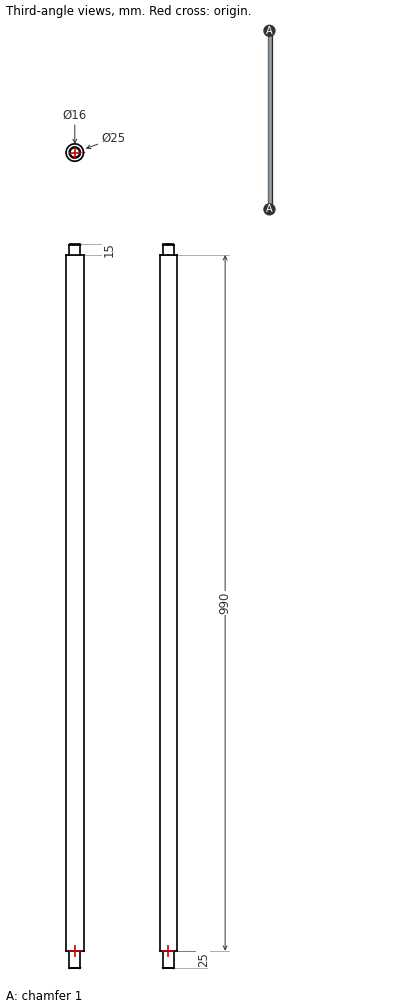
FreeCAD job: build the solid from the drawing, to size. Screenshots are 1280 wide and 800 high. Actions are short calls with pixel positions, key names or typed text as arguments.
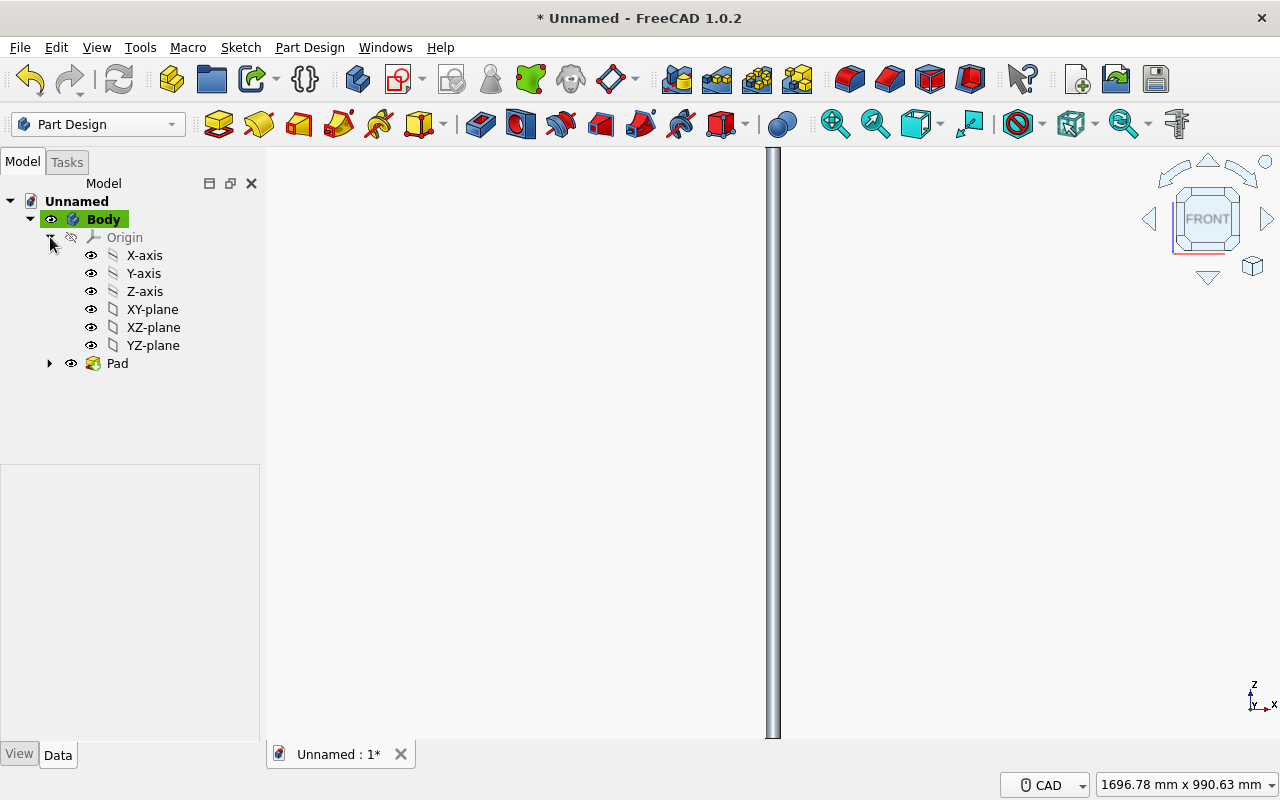
click(136, 309)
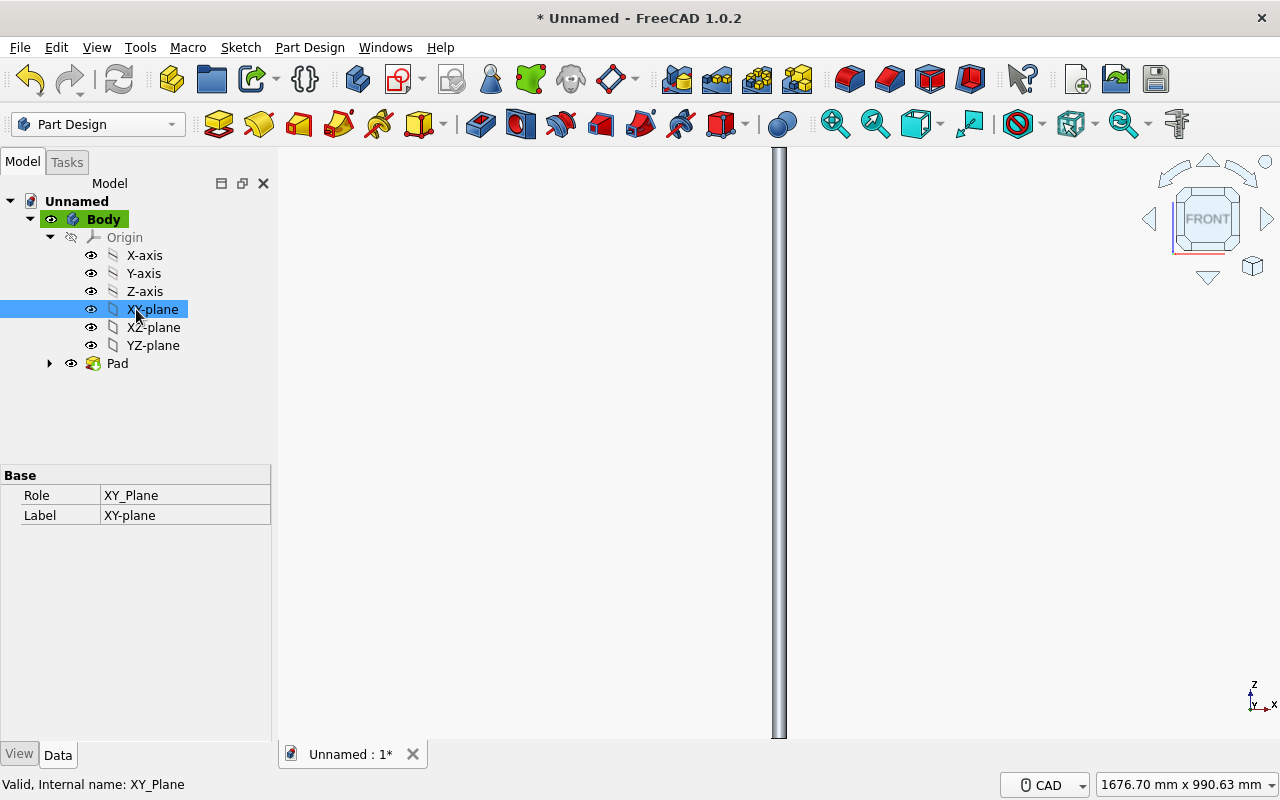
click(612, 80)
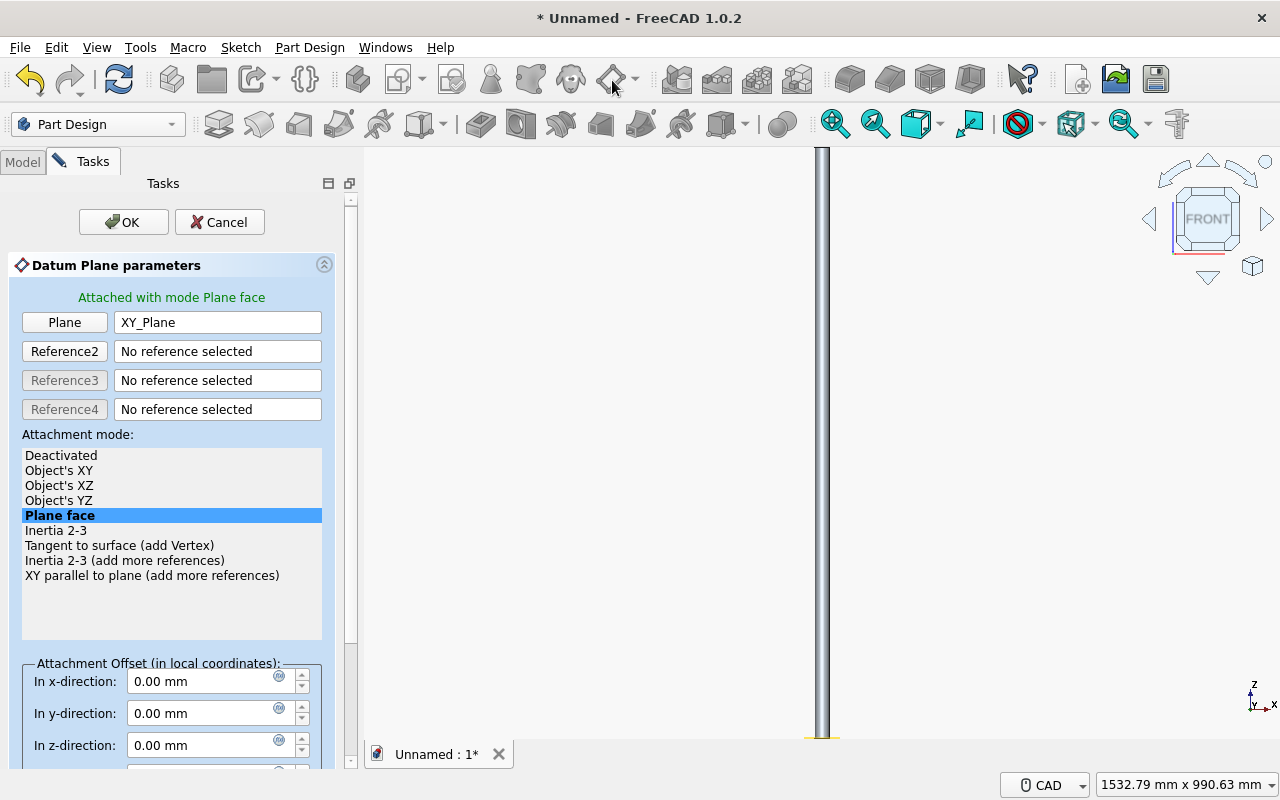
triple_click(210, 745)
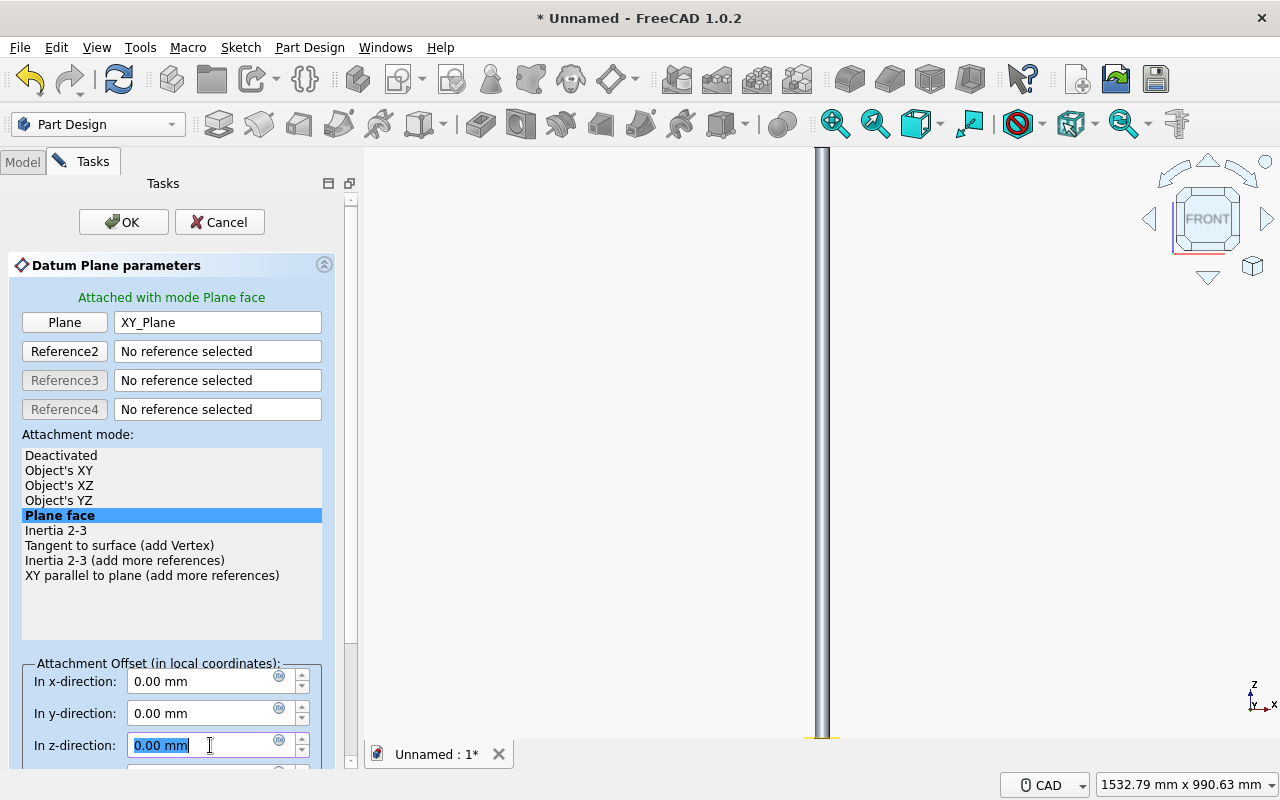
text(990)
key(Tab)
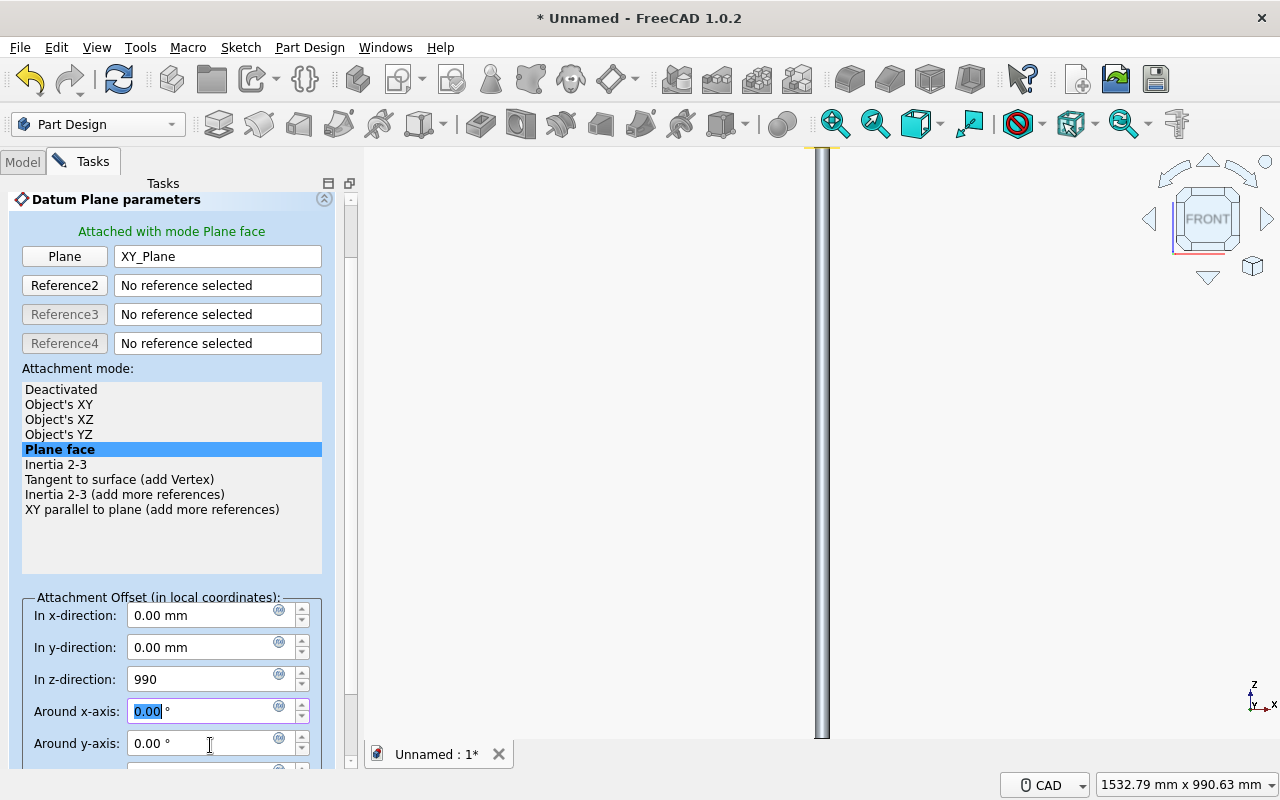
scroll(351, 480, up, 2)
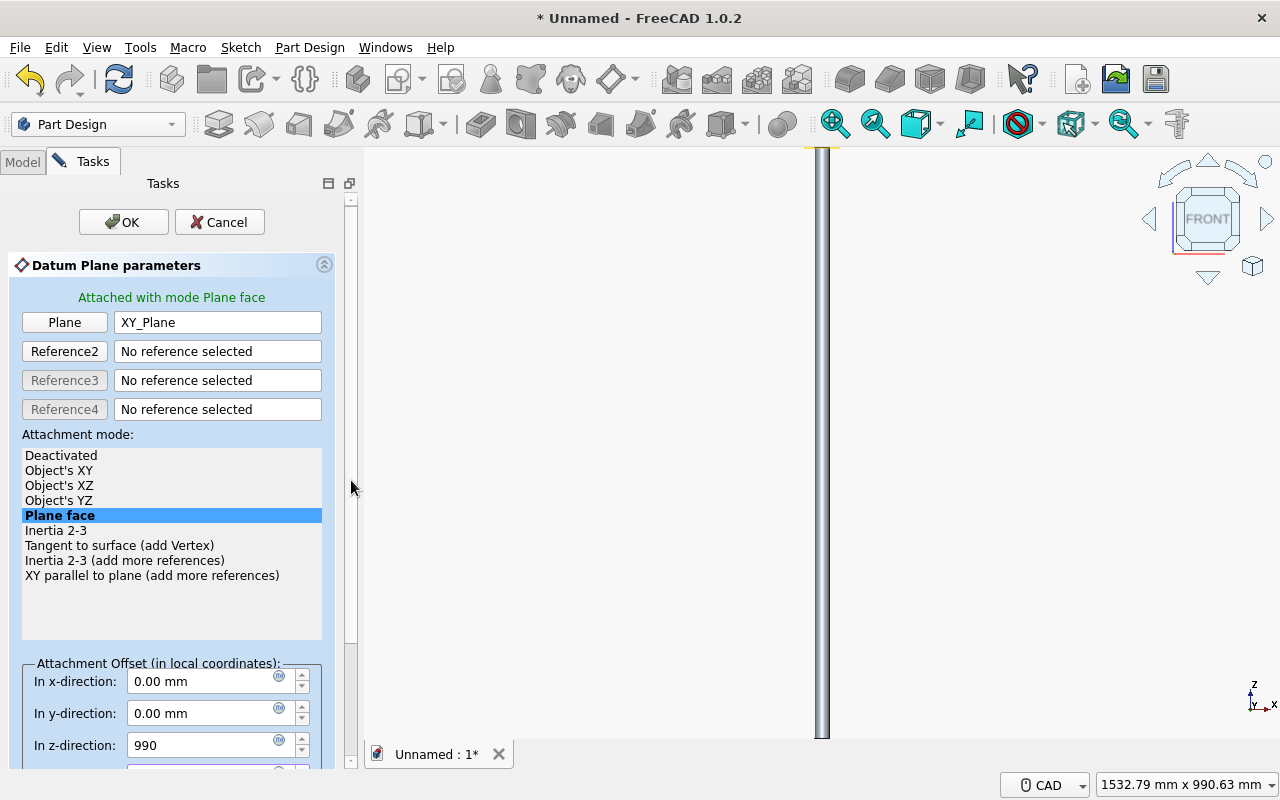
click(124, 222)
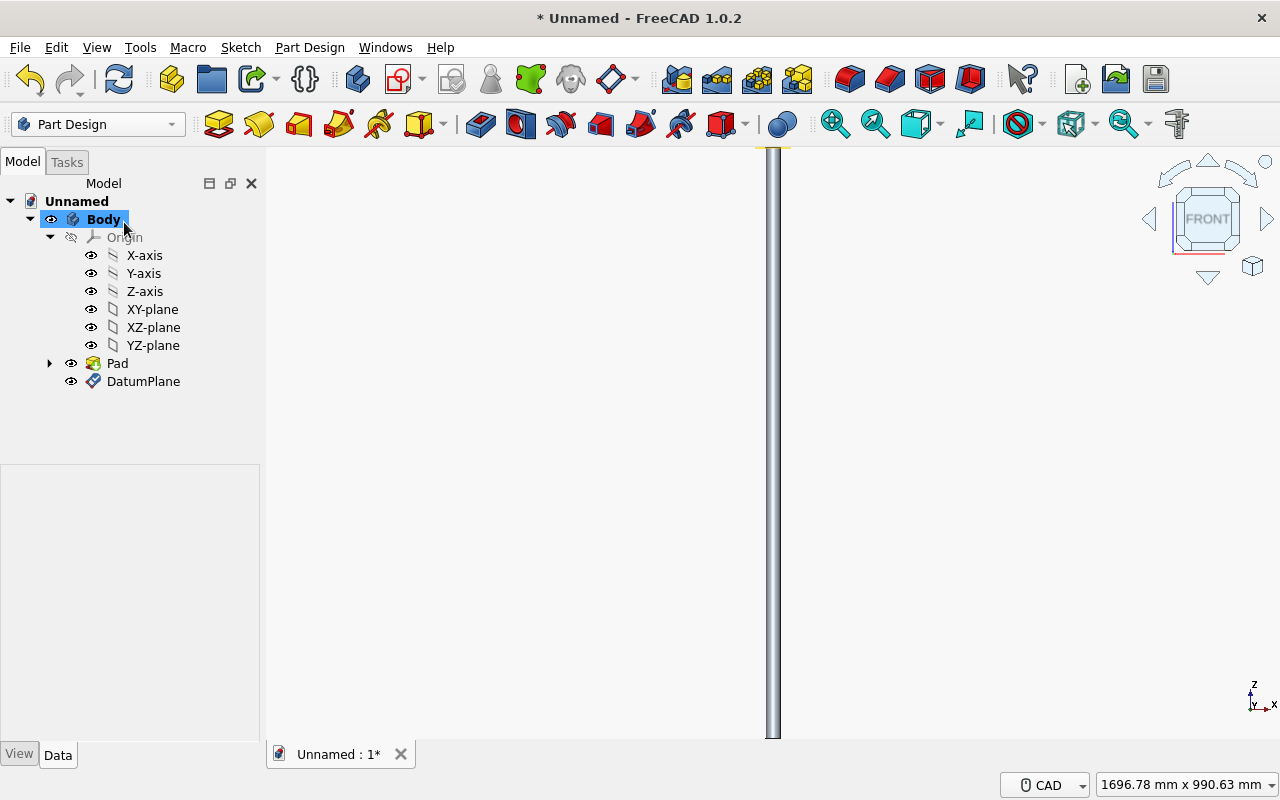
click(116, 381)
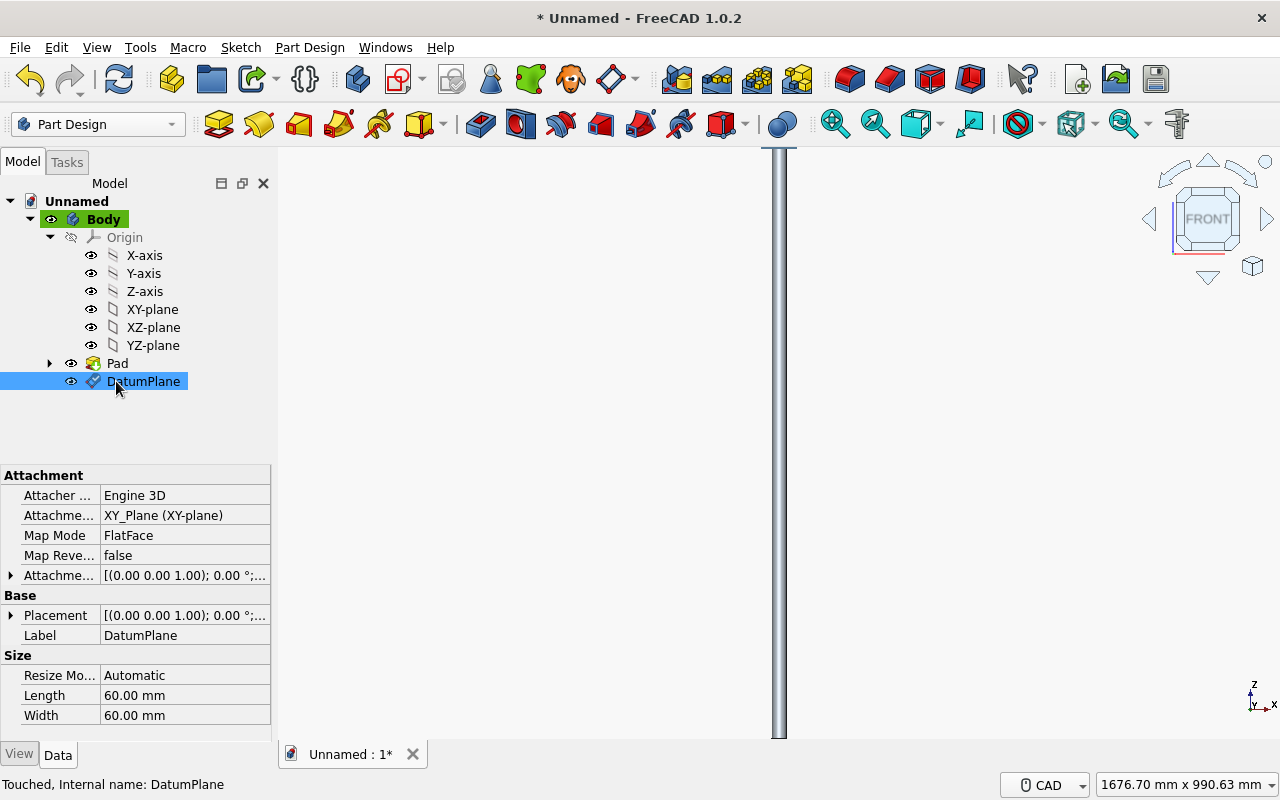
click(398, 80)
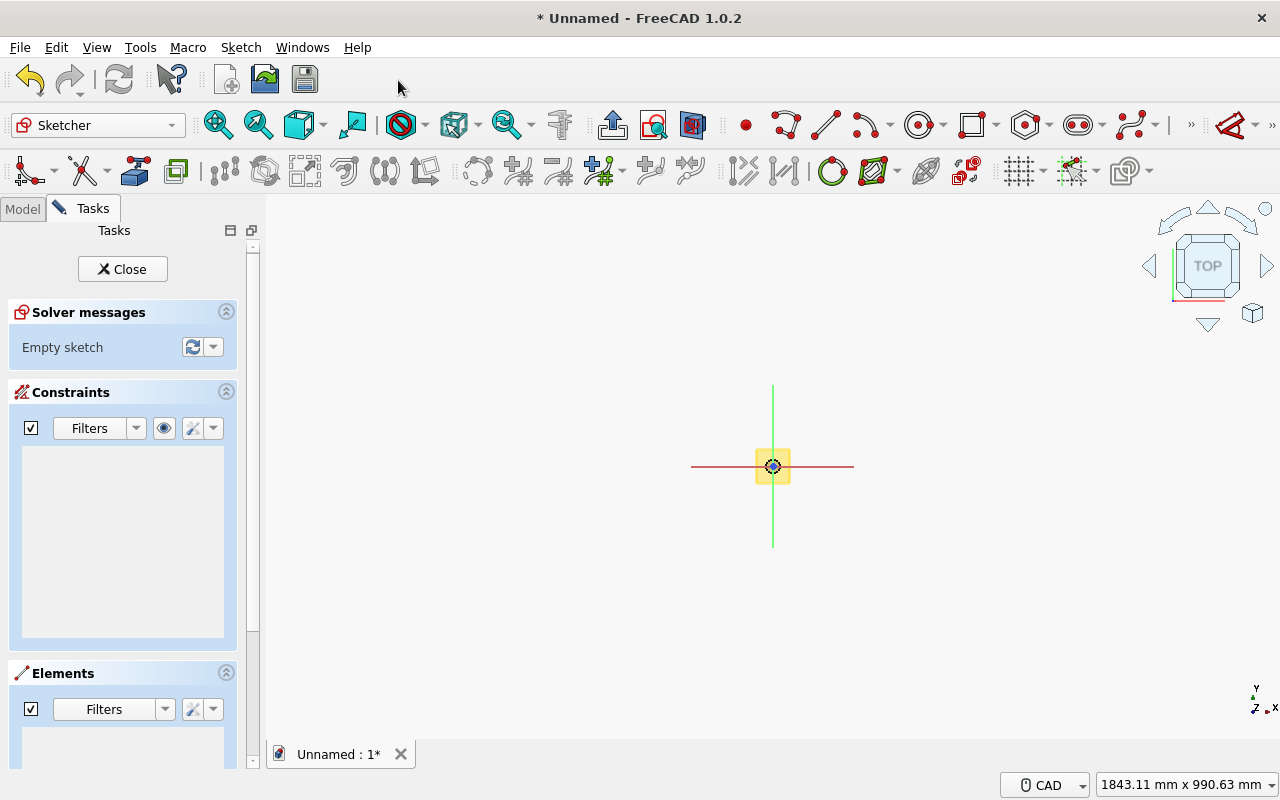
scroll(777, 466, up, 15)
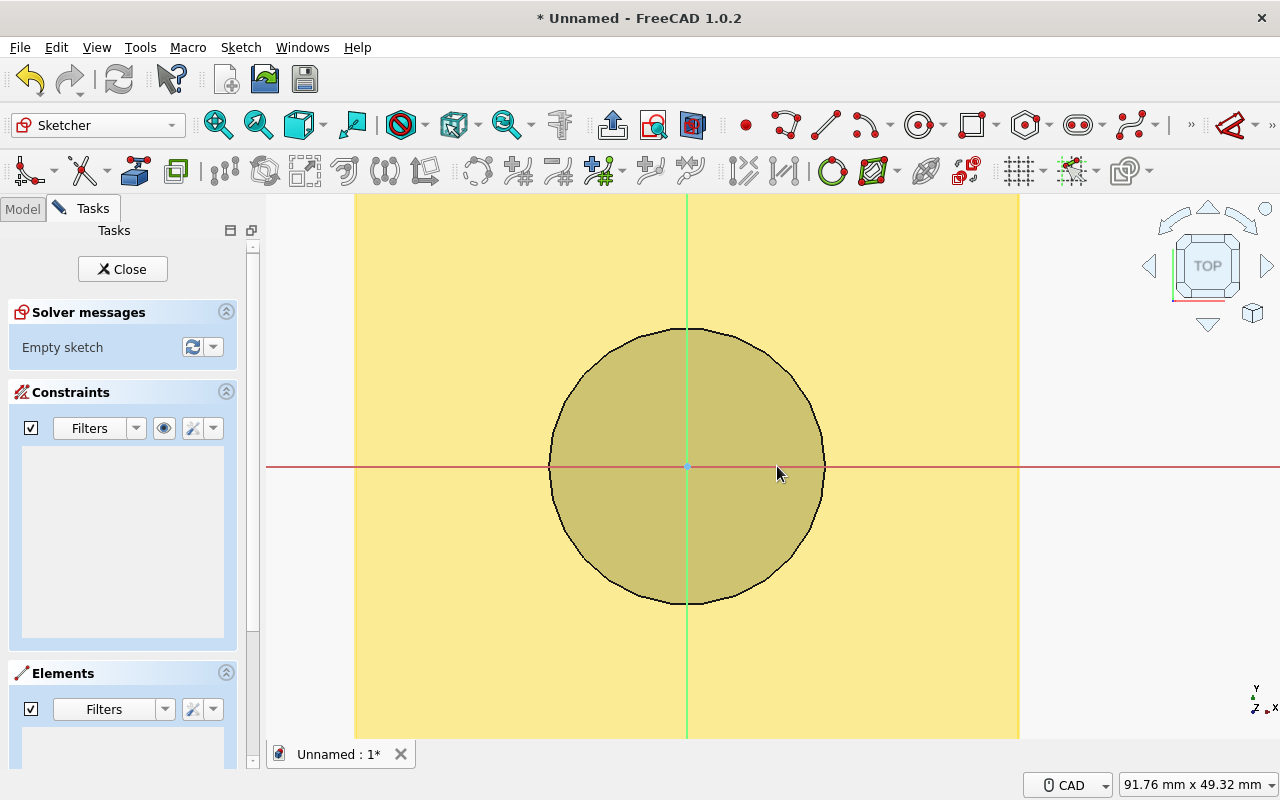
scroll(666, 466, up, 3)